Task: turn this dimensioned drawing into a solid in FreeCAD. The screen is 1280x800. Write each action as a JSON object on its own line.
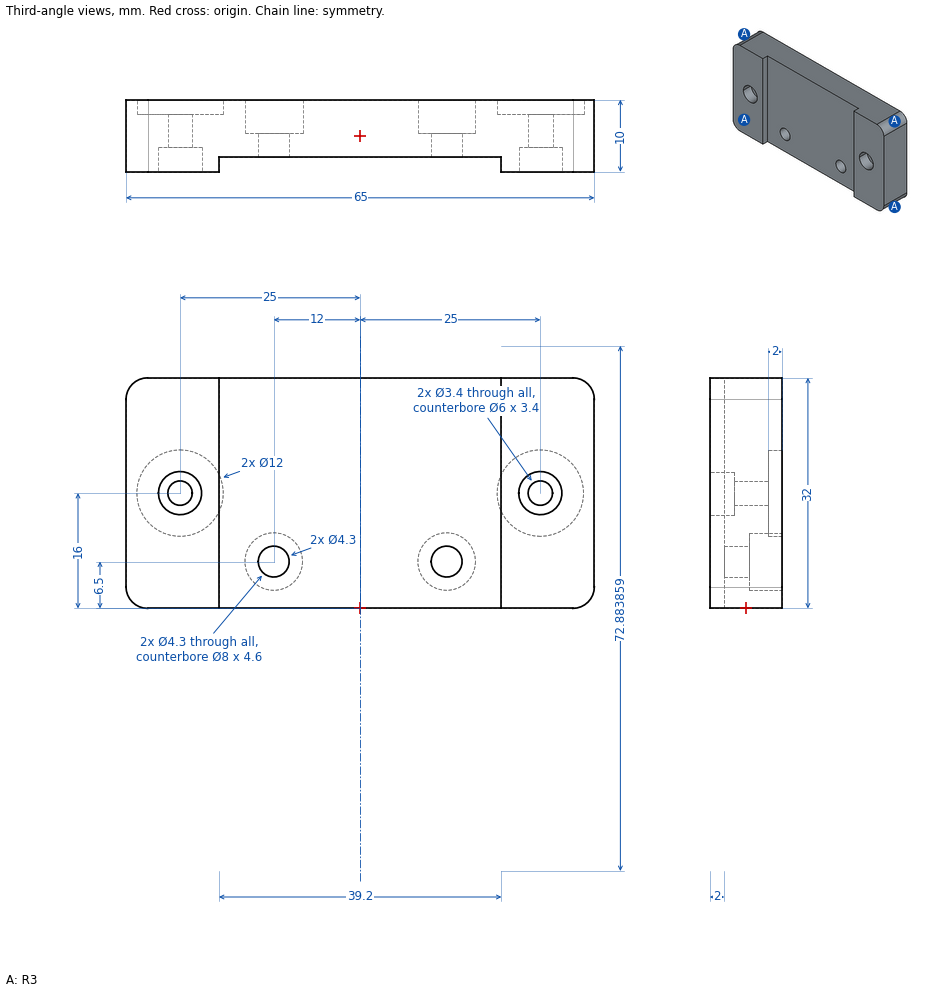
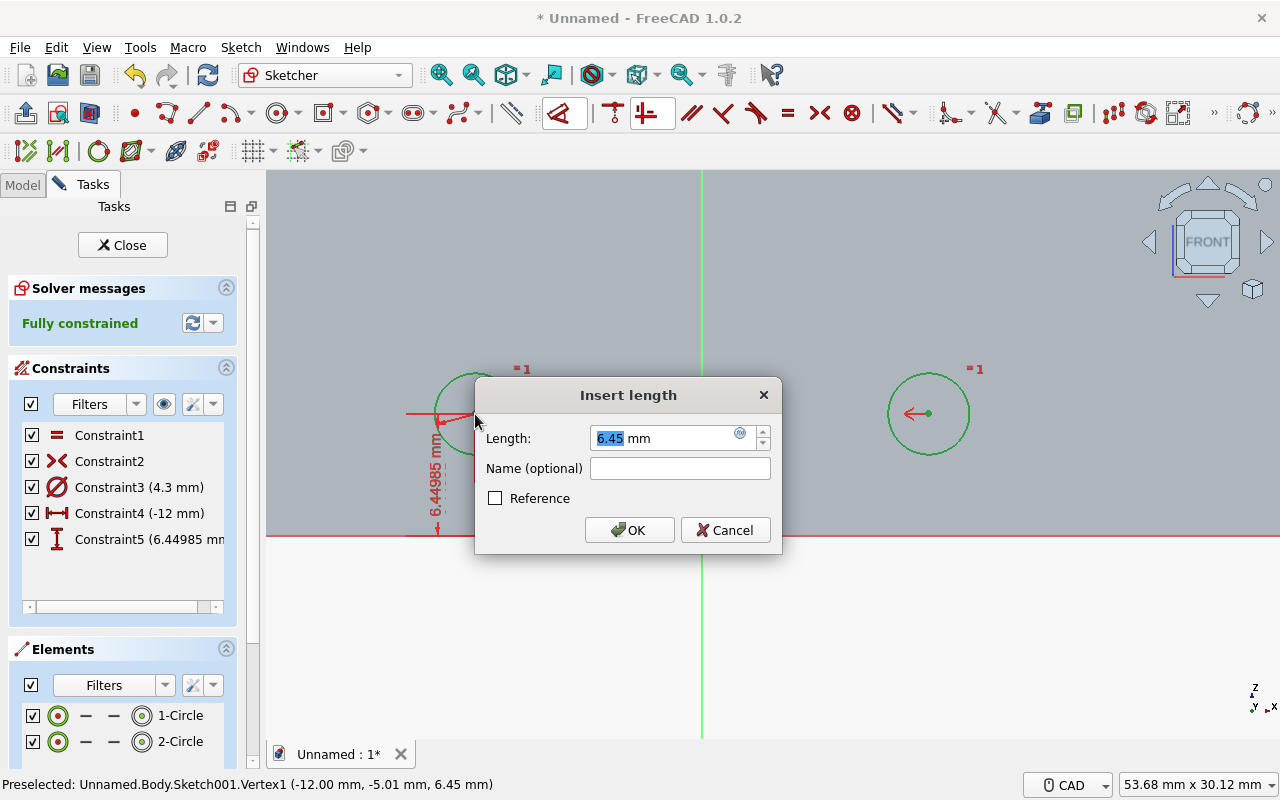
{"action": "type", "text": "6.5"}
{"action": "key", "text": "Return"}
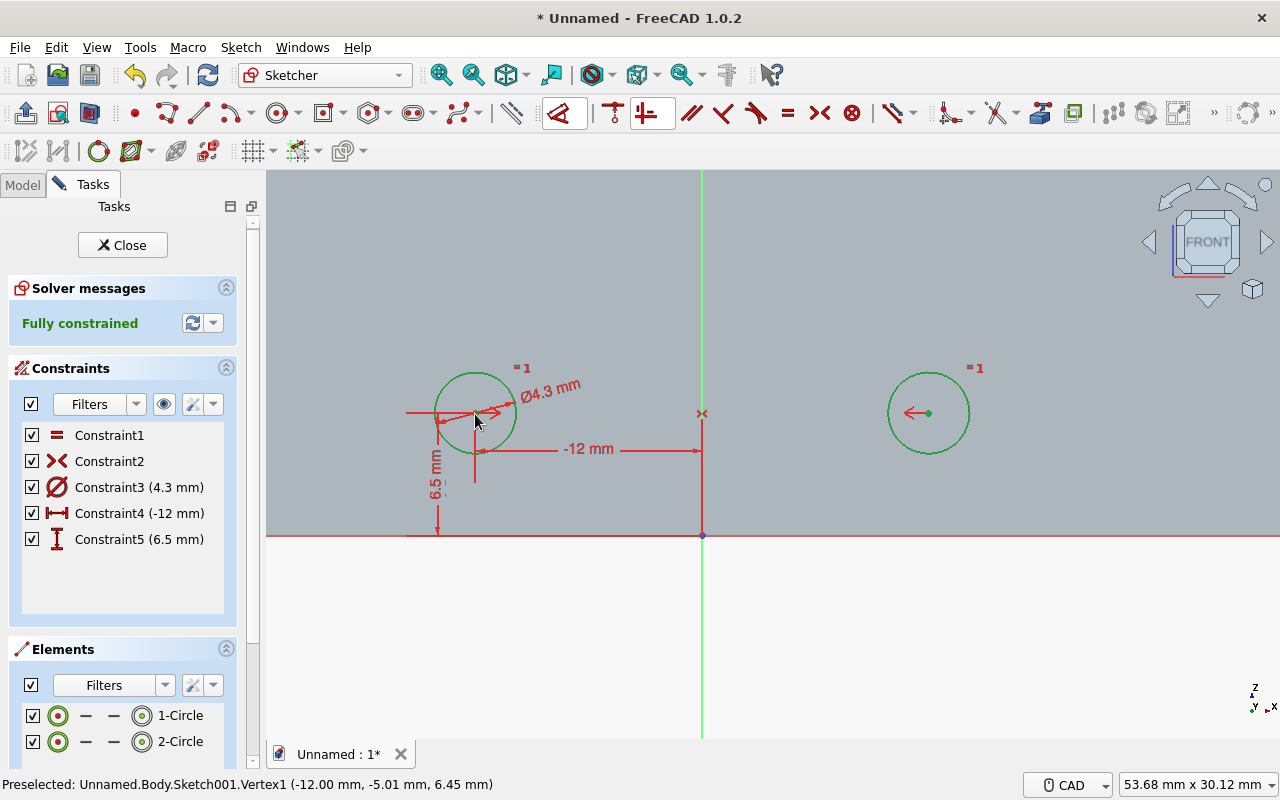
{"action": "left_click", "coordinate": [123, 245]}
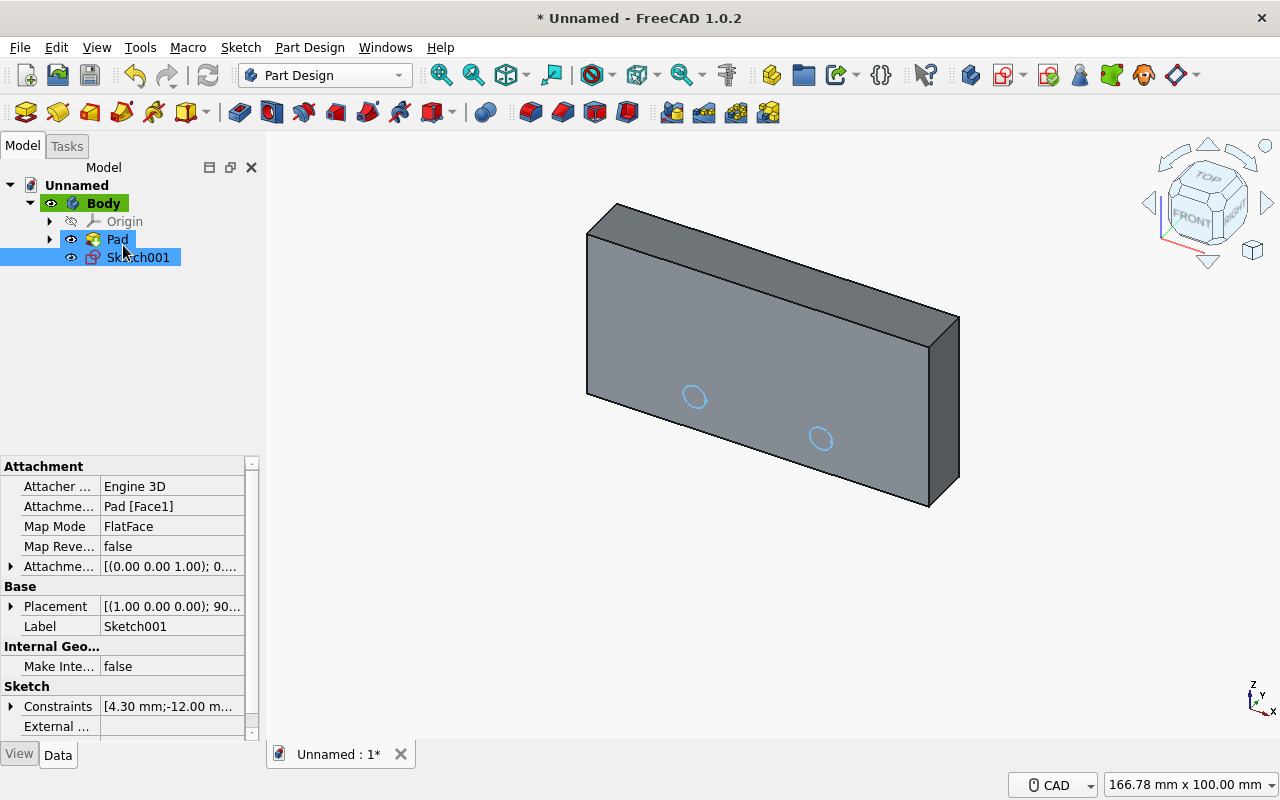
{"action": "left_click", "coordinate": [240, 112]}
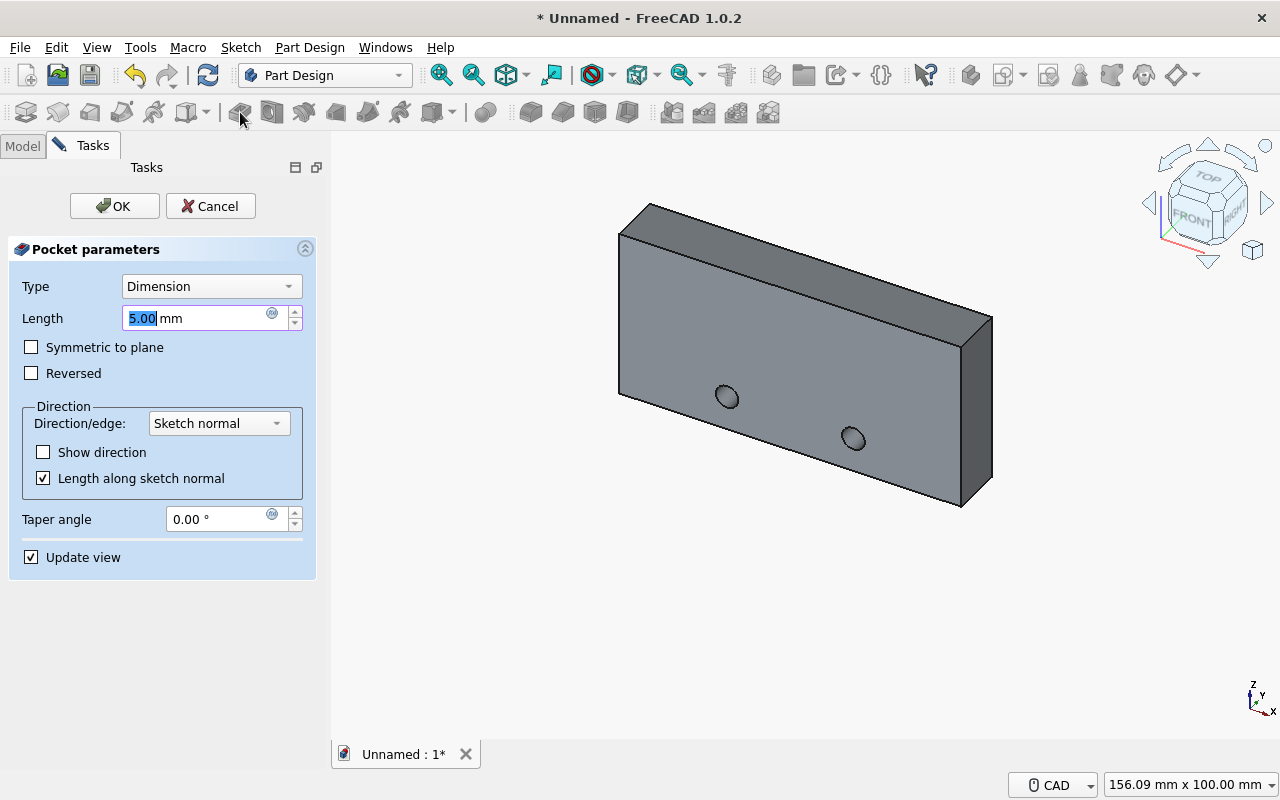
{"action": "left_click", "coordinate": [212, 286]}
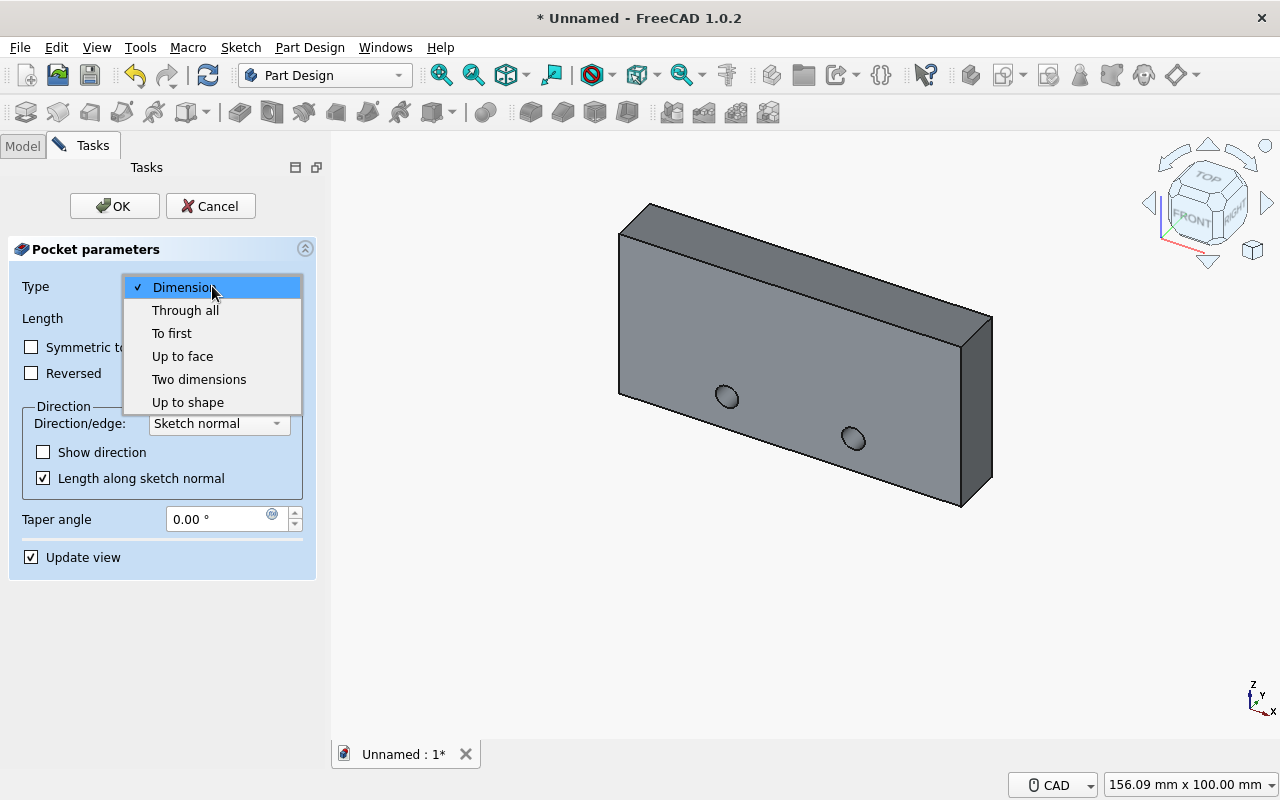
{"action": "left_click", "coordinate": [212, 310]}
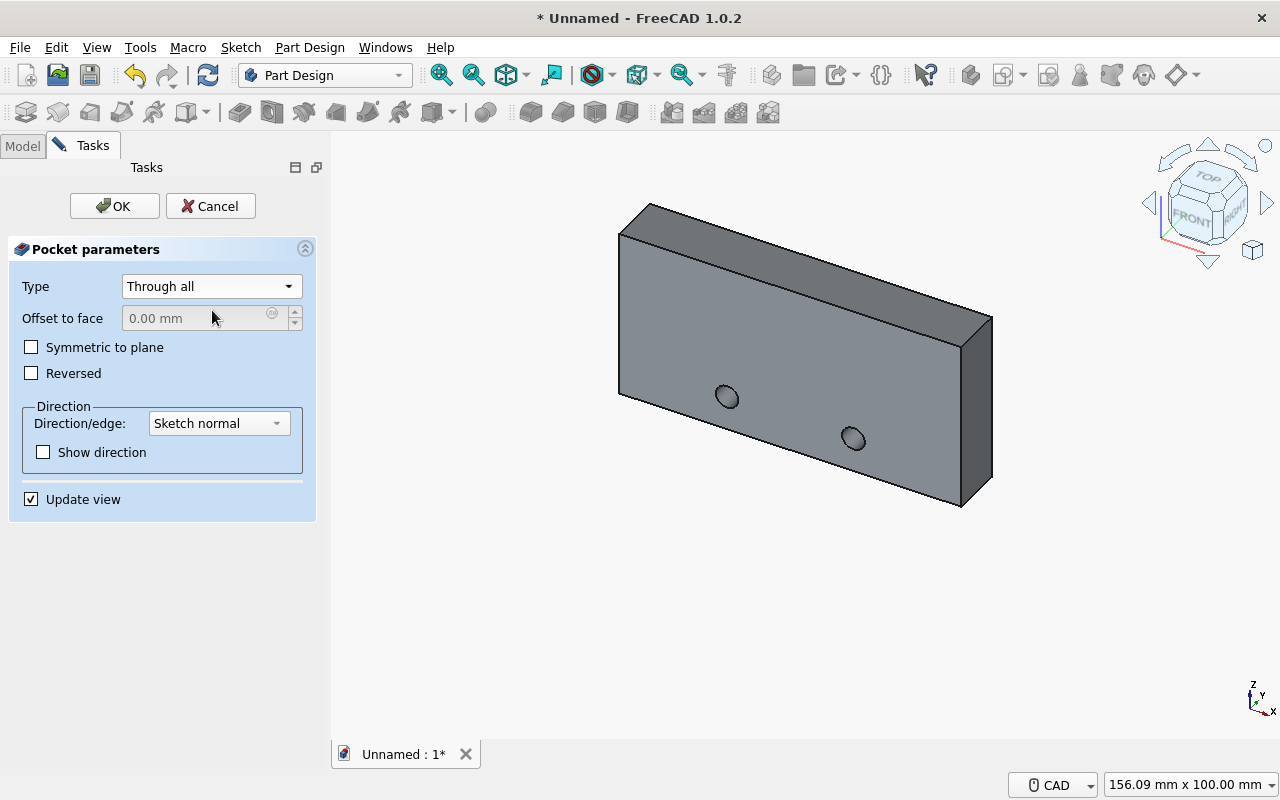
{"action": "left_click", "coordinate": [115, 206]}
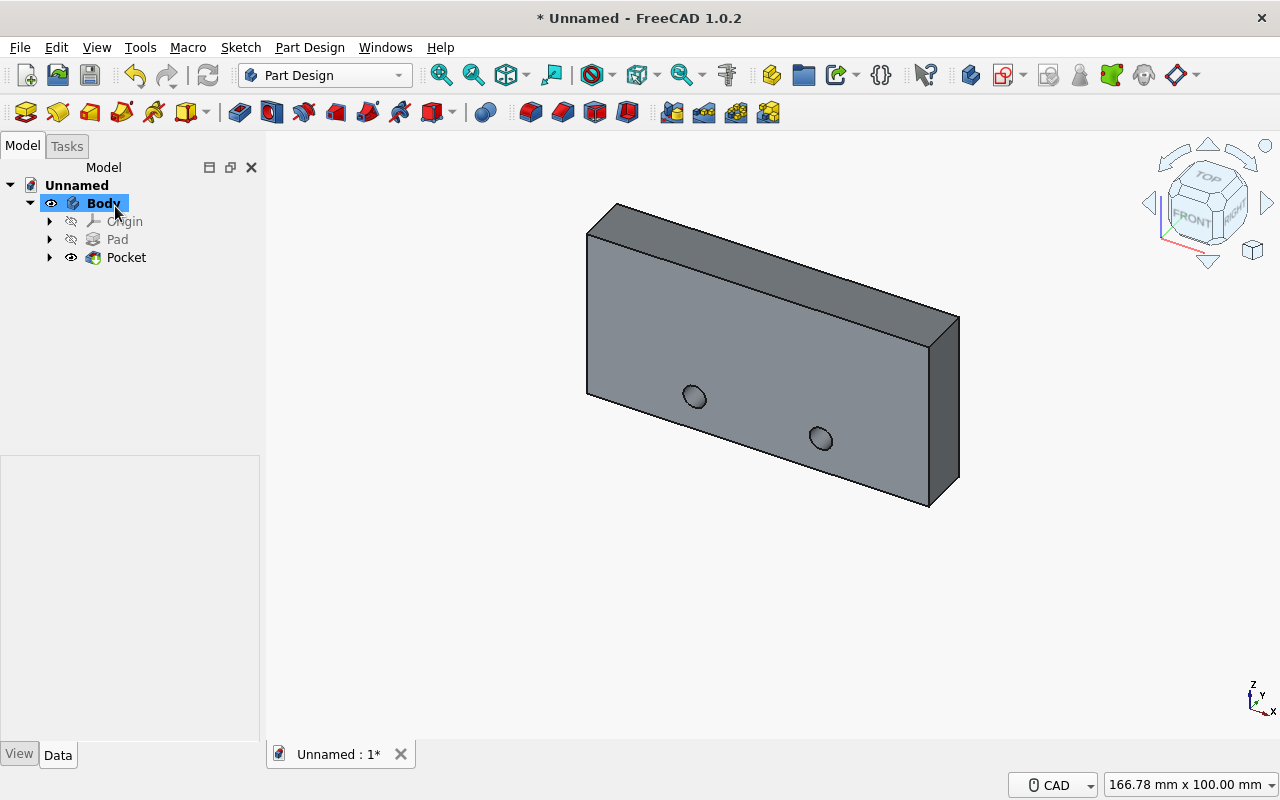
{"action": "left_click", "coordinate": [944, 331]}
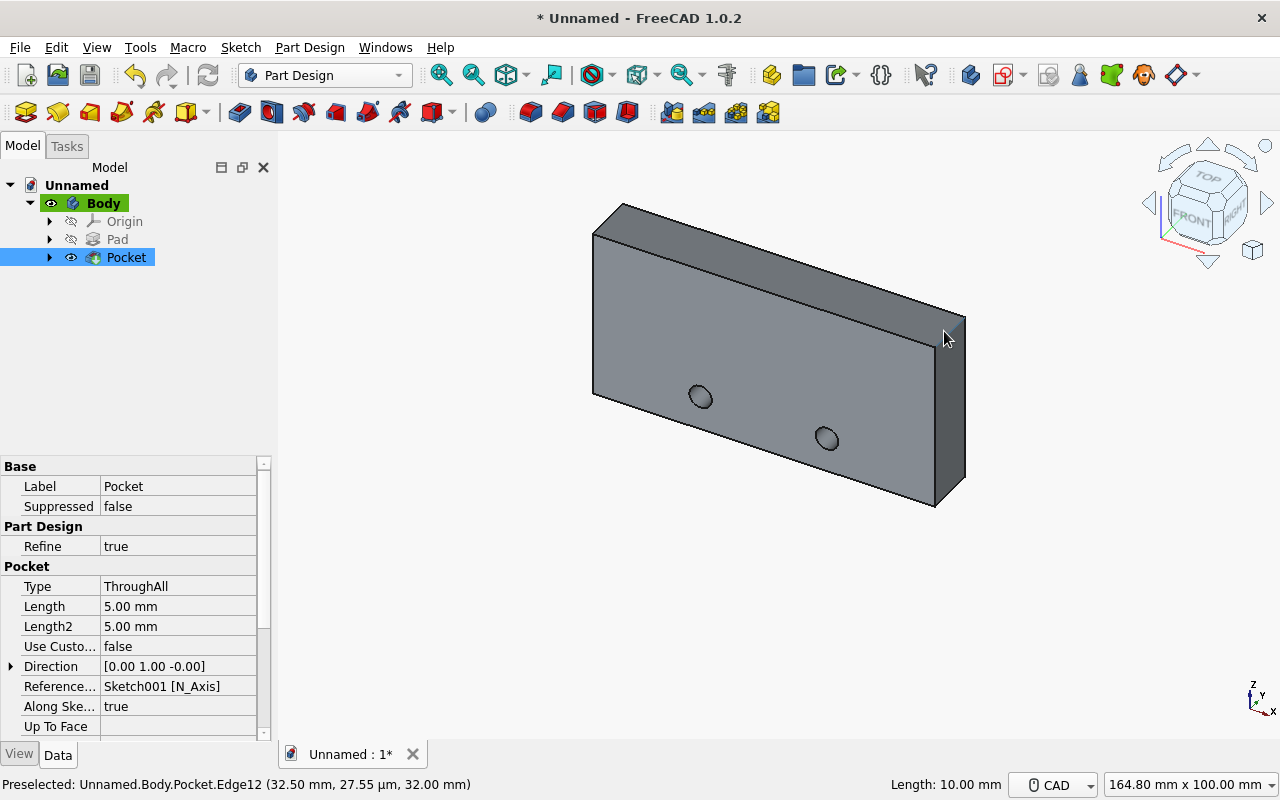
{"action": "key", "text": "0"}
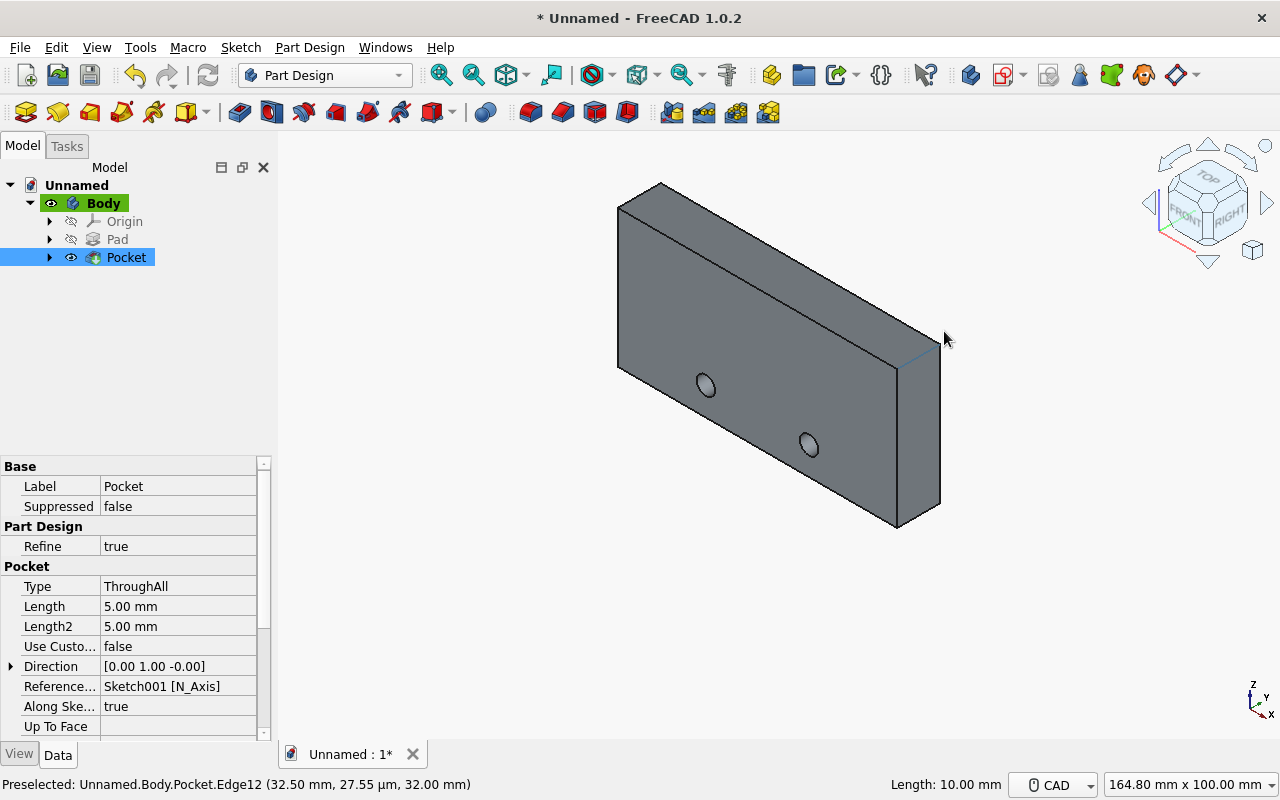
{"action": "key", "text": "2"}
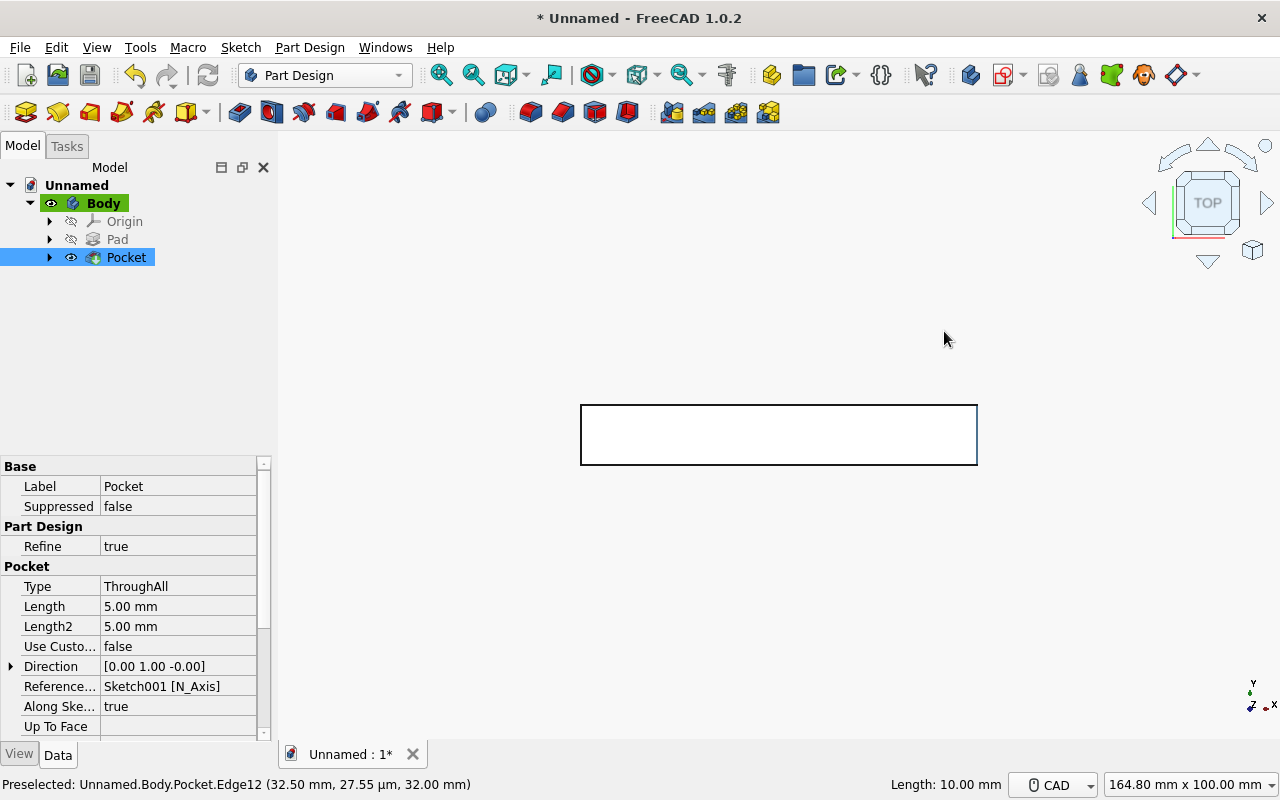
{"action": "left_click", "coordinate": [442, 76]}